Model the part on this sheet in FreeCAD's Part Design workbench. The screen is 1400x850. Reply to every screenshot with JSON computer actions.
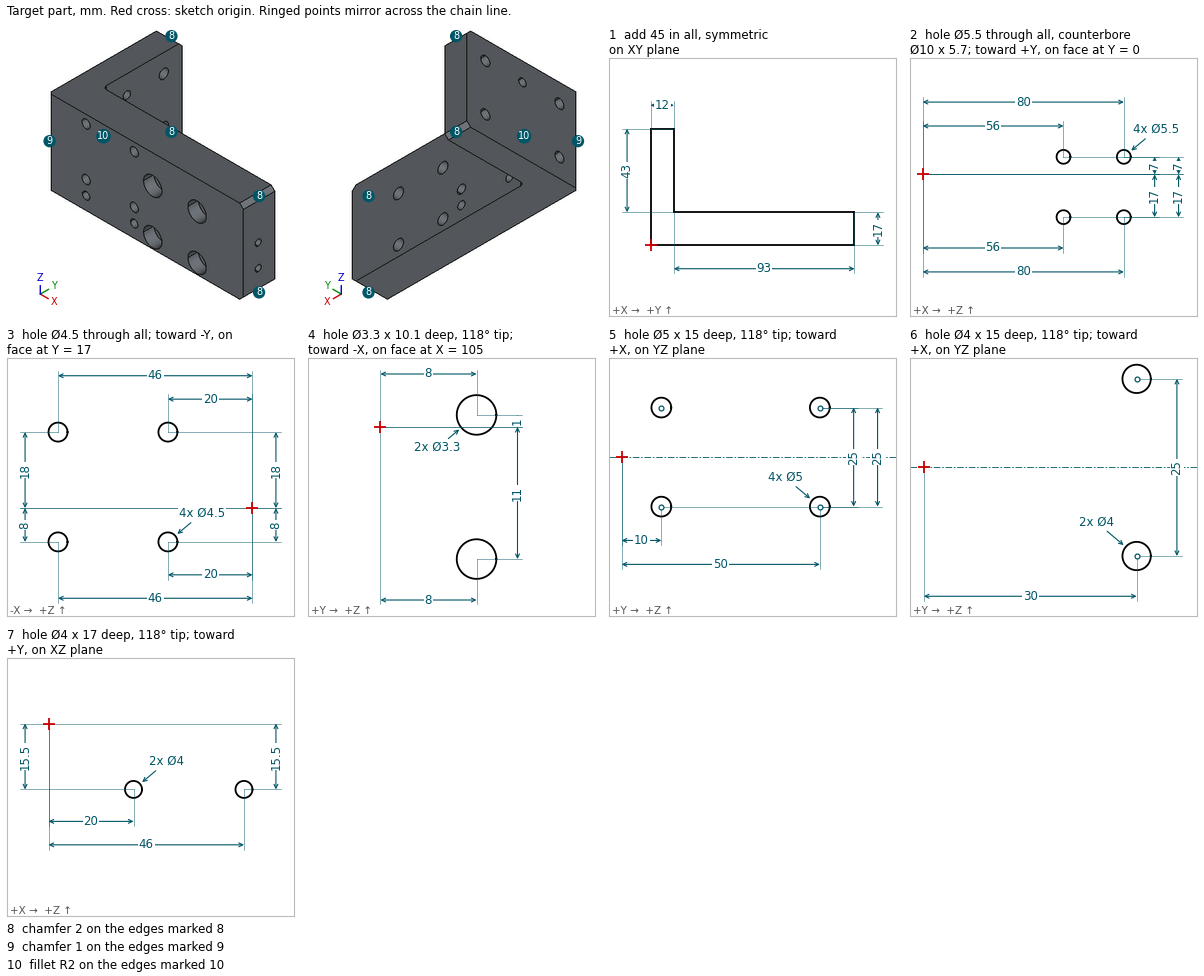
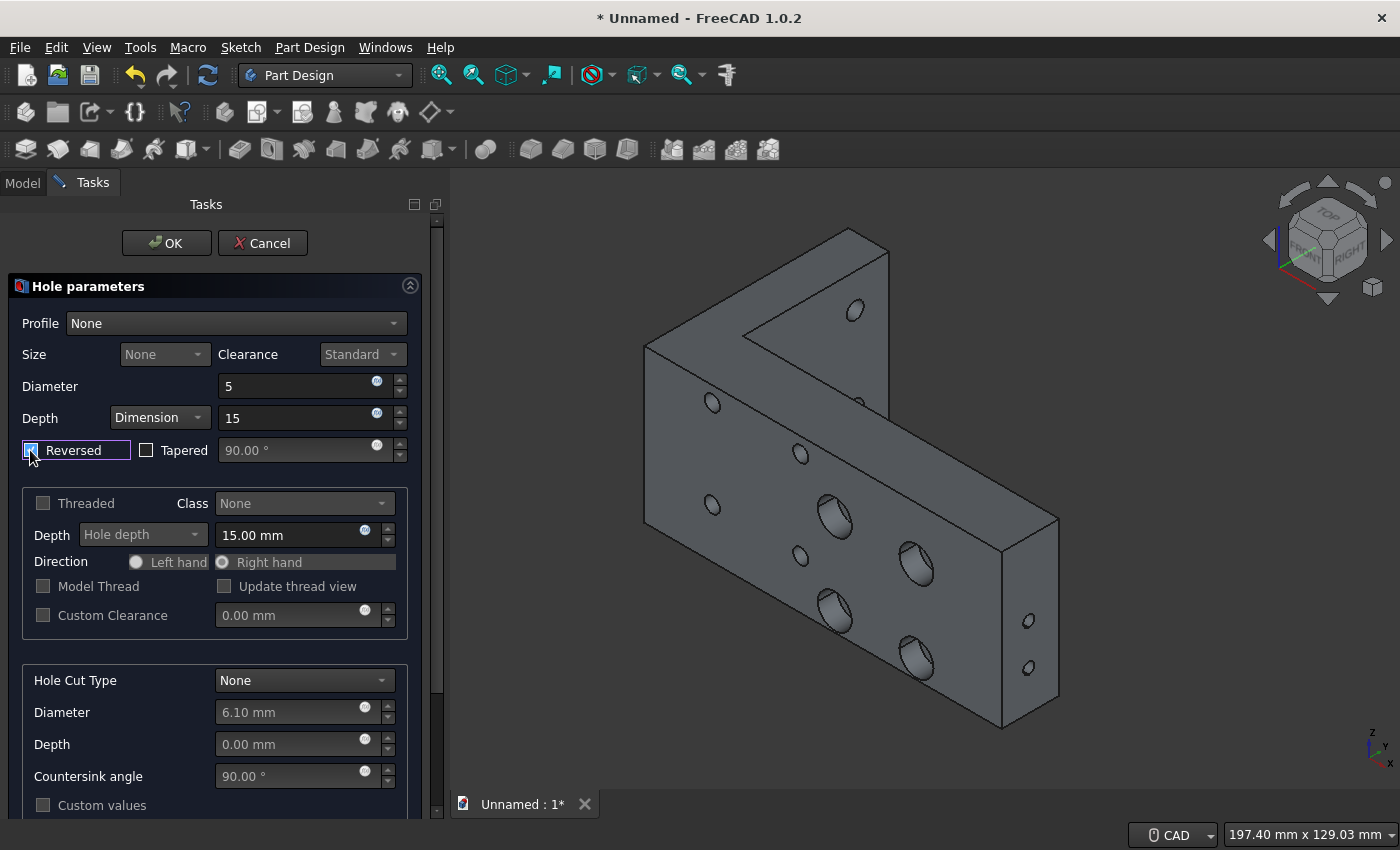
{"action": "left_click", "coordinate": [167, 243]}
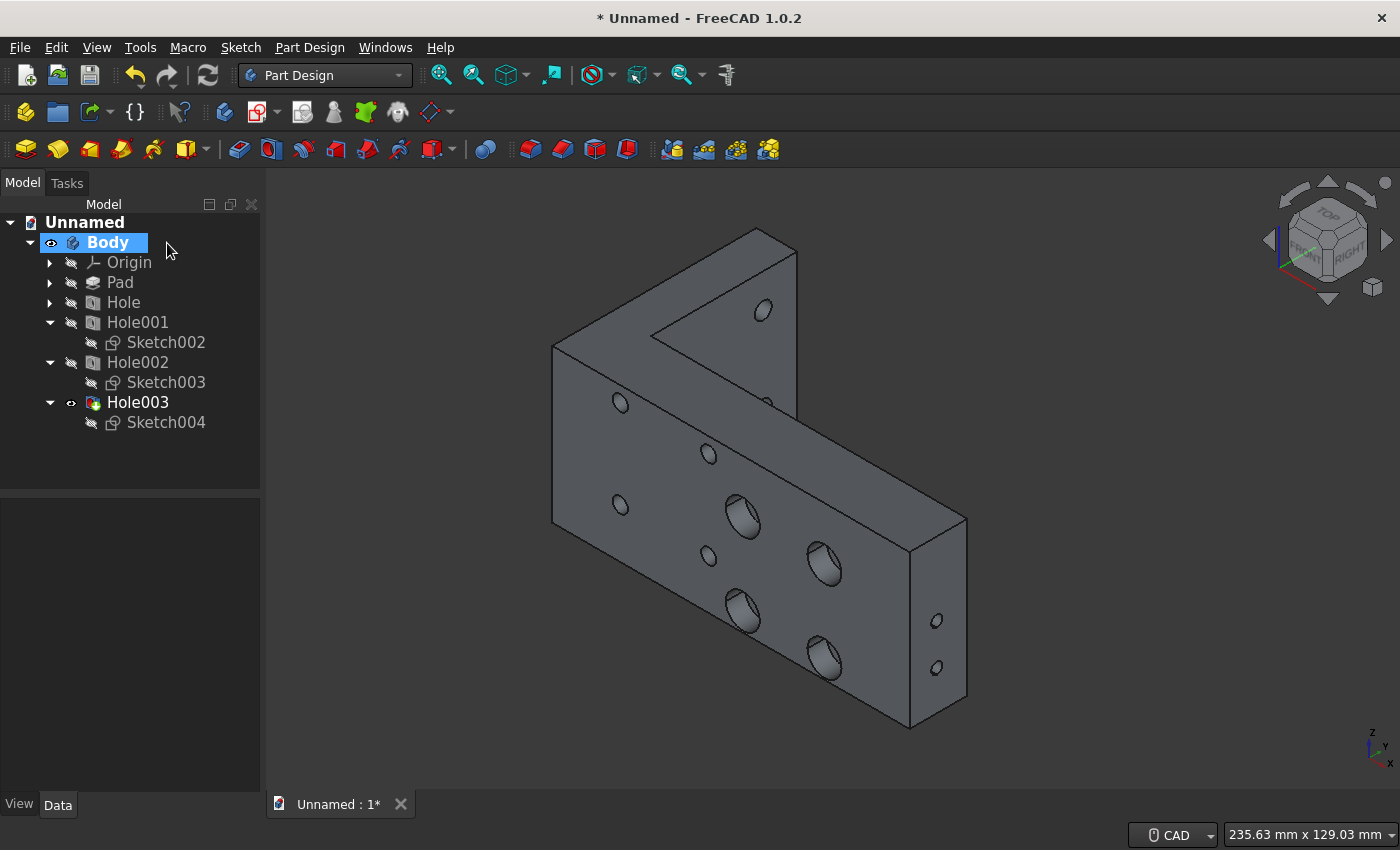
{"action": "left_click", "coordinate": [258, 112]}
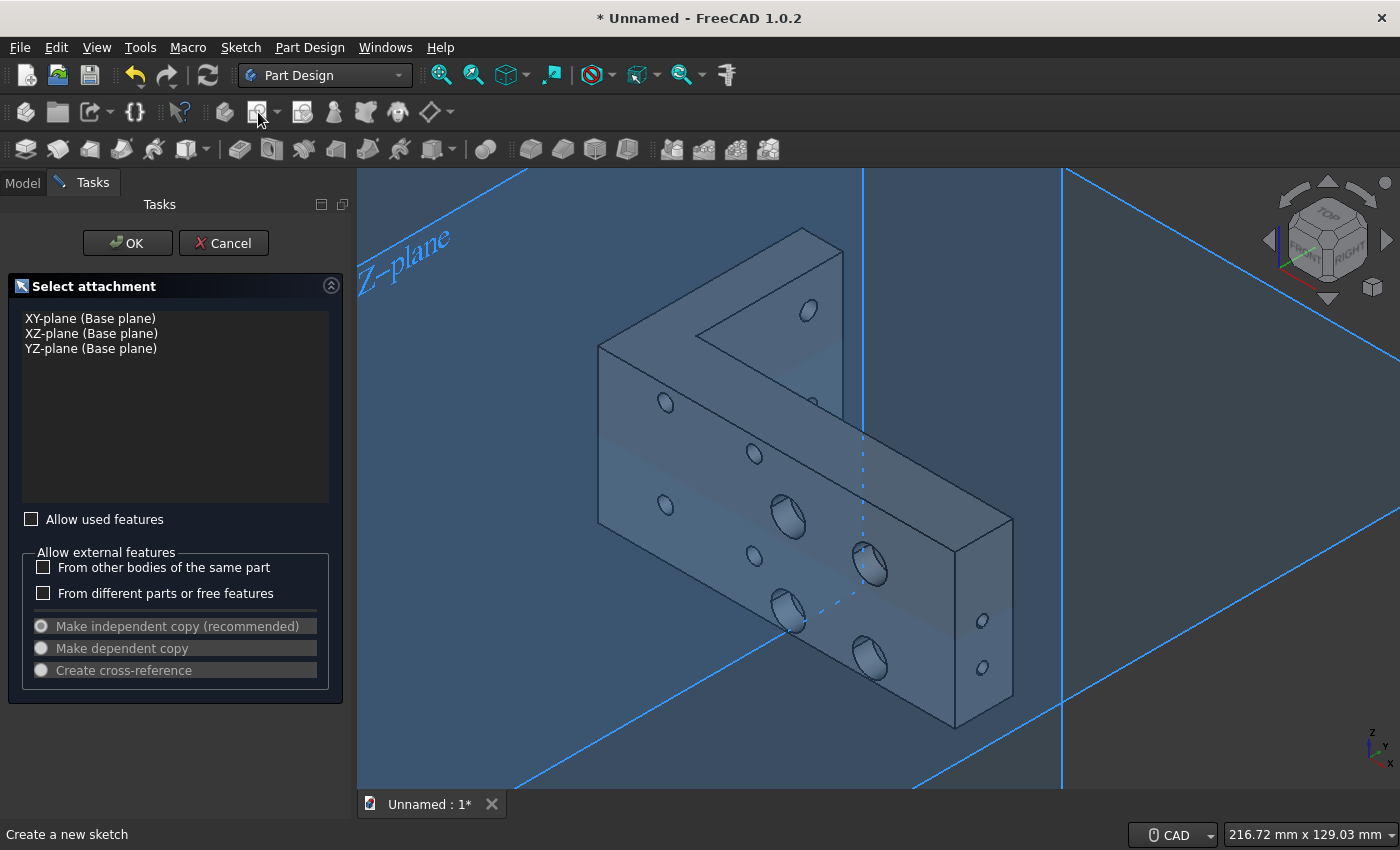
{"action": "left_click", "coordinate": [82, 348]}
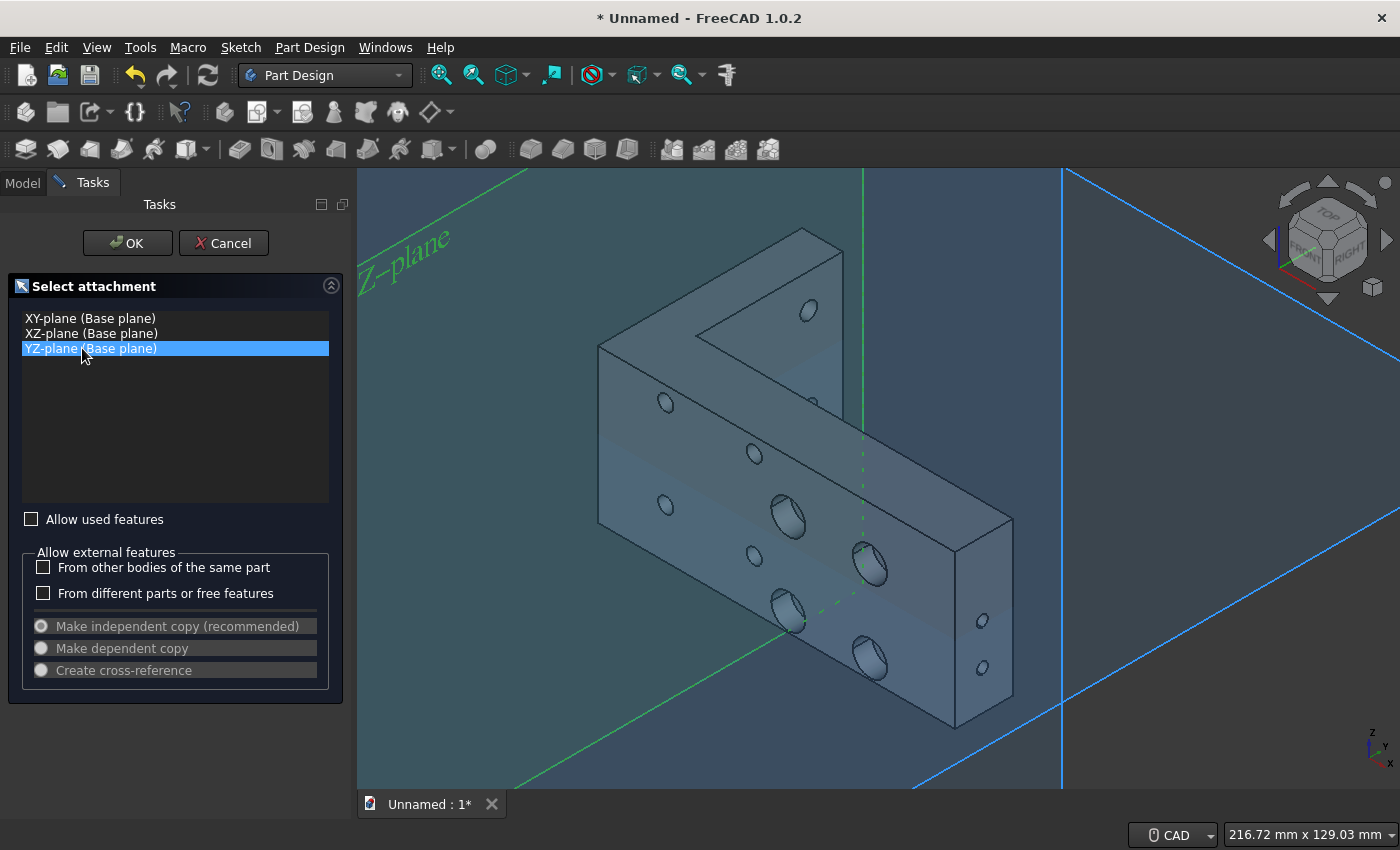
{"action": "left_click", "coordinate": [128, 243]}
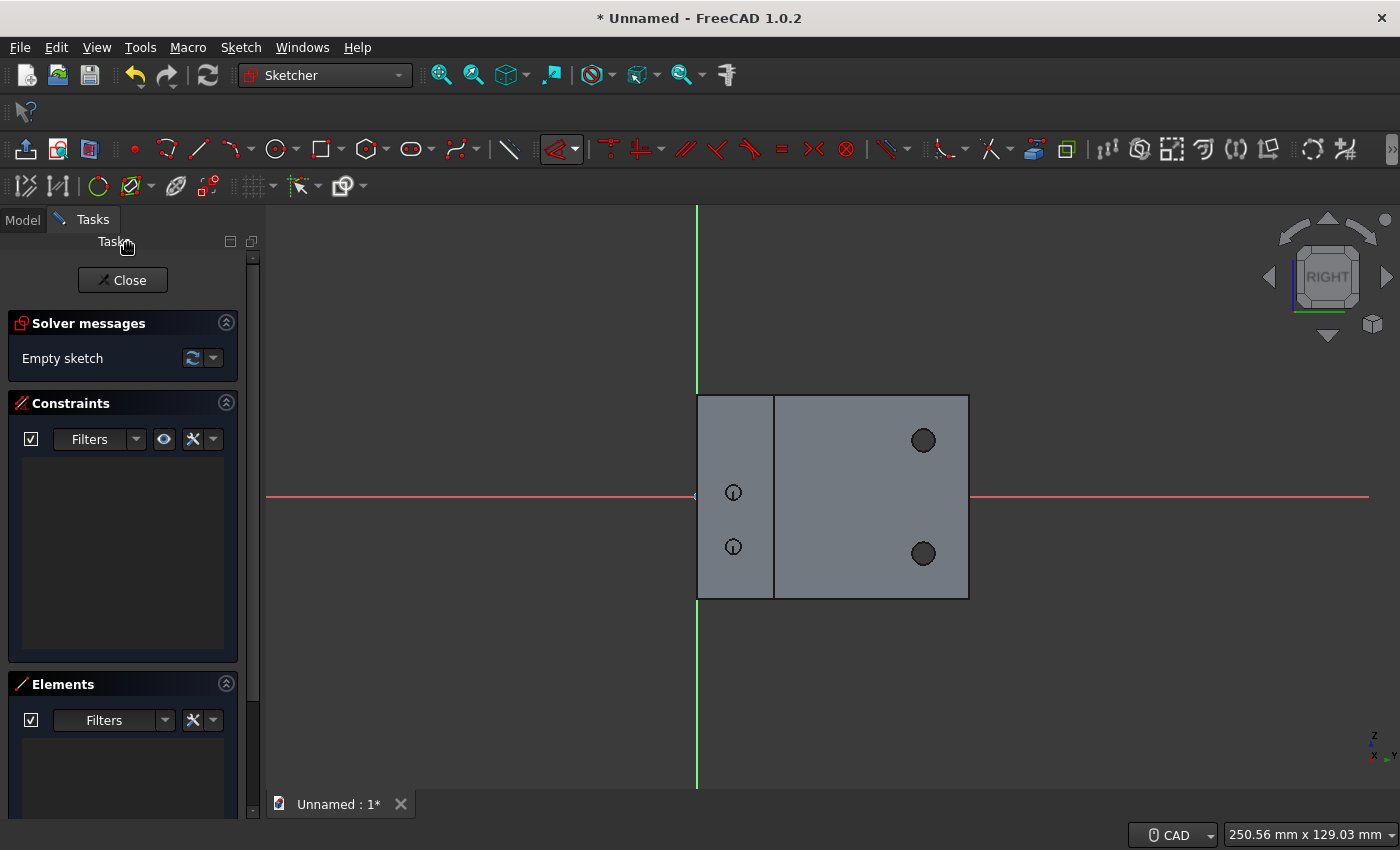
{"action": "key", "text": "q s"}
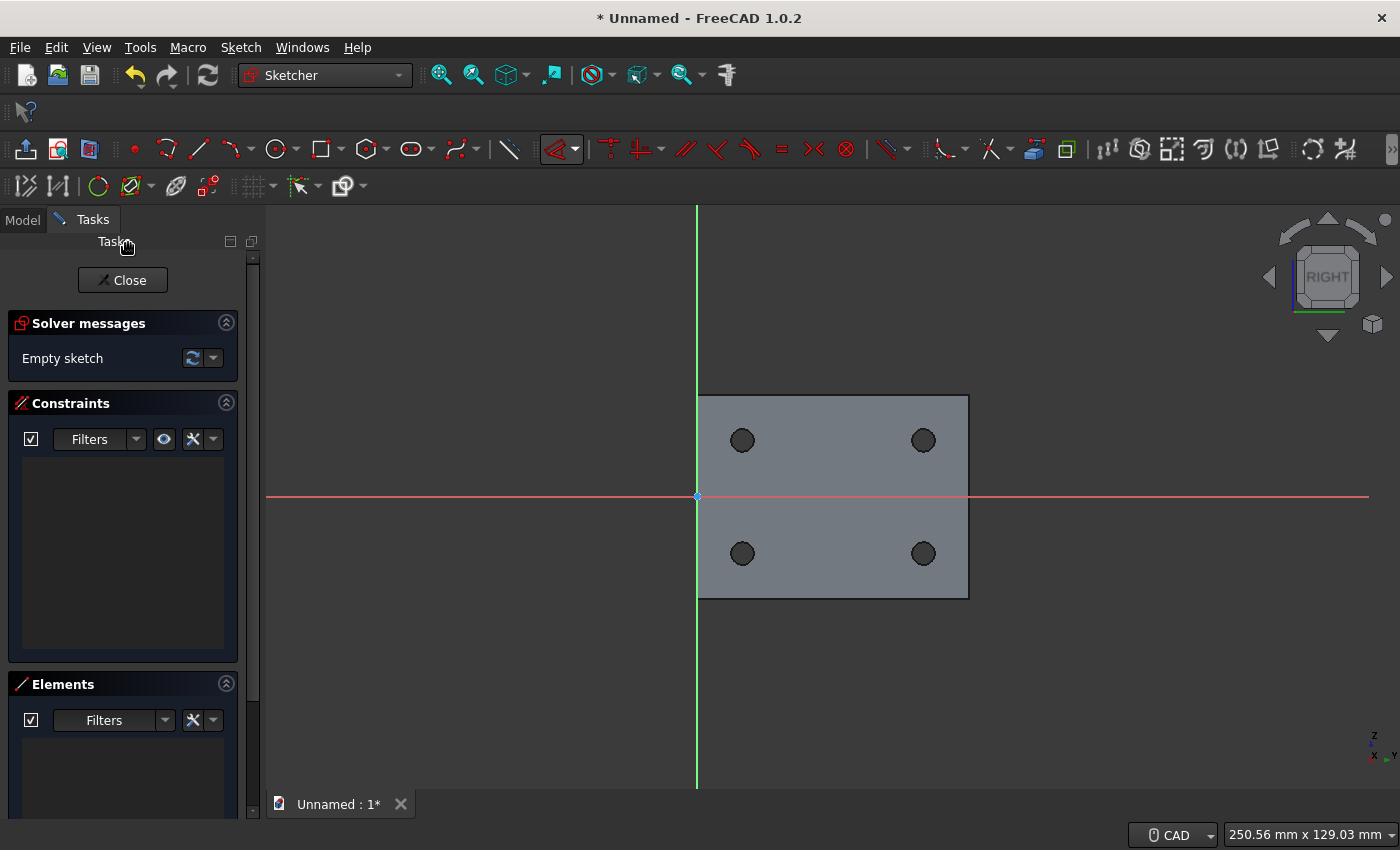
{"action": "scroll", "coordinate": [773, 497], "scroll_direction": "up", "scroll_amount": 5}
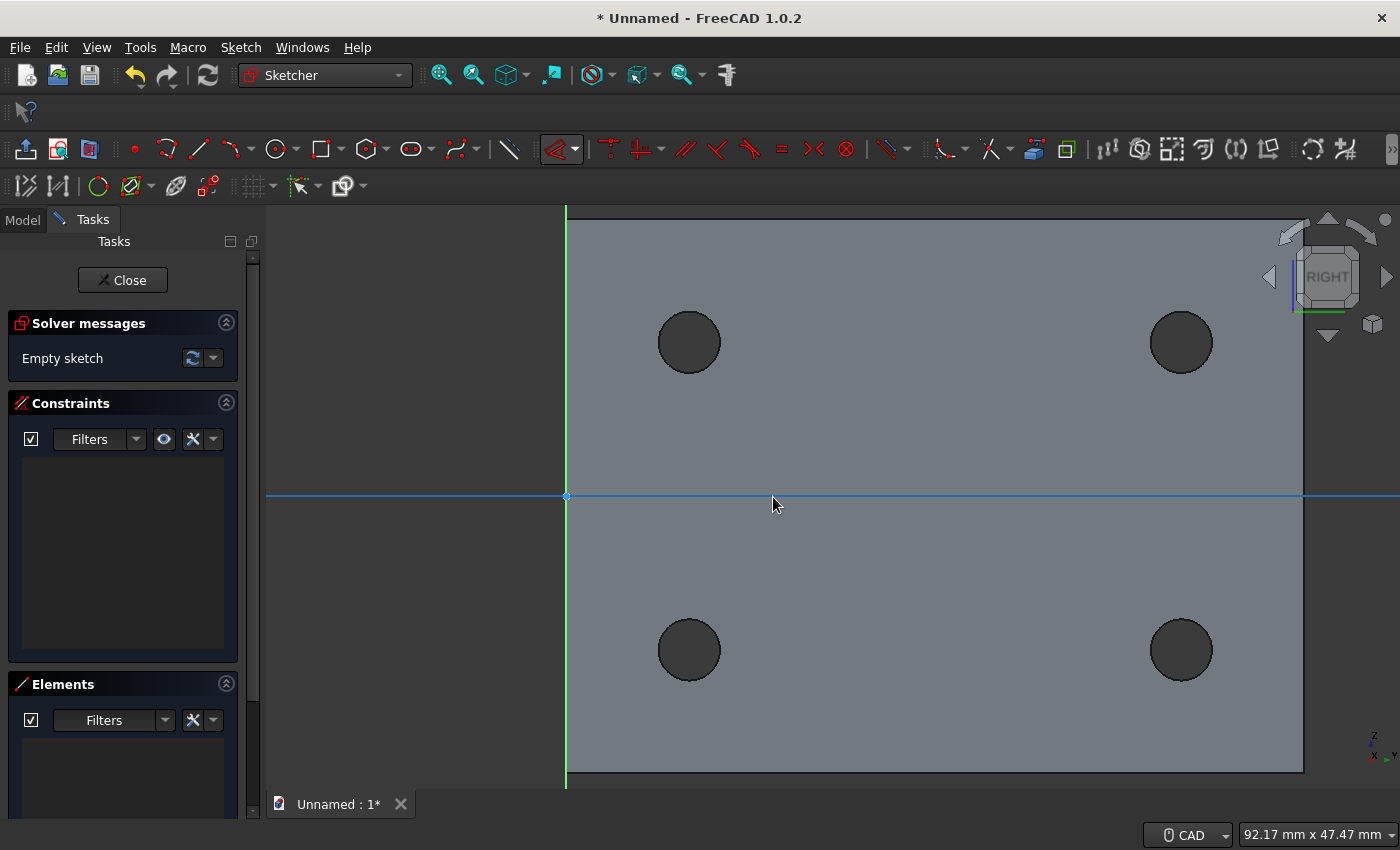
{"action": "key", "text": "g c"}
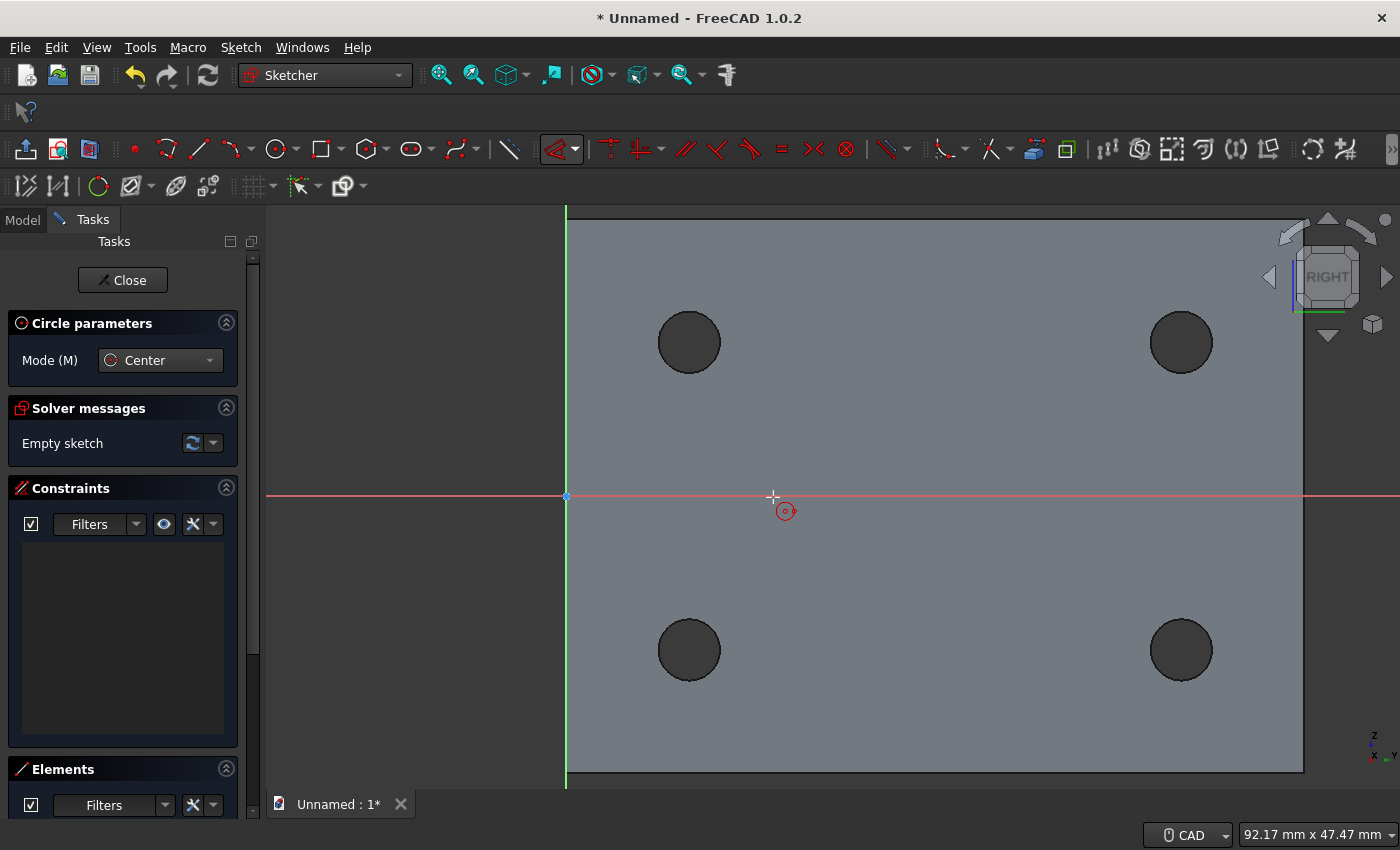
{"action": "left_click", "coordinate": [935, 650]}
{"action": "left_click", "coordinate": [953, 633]}